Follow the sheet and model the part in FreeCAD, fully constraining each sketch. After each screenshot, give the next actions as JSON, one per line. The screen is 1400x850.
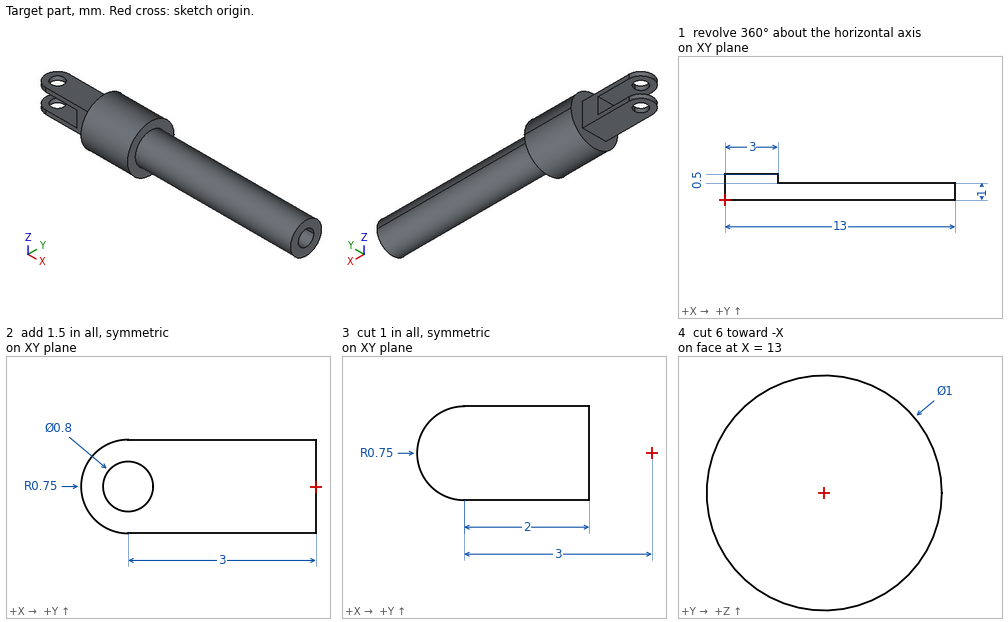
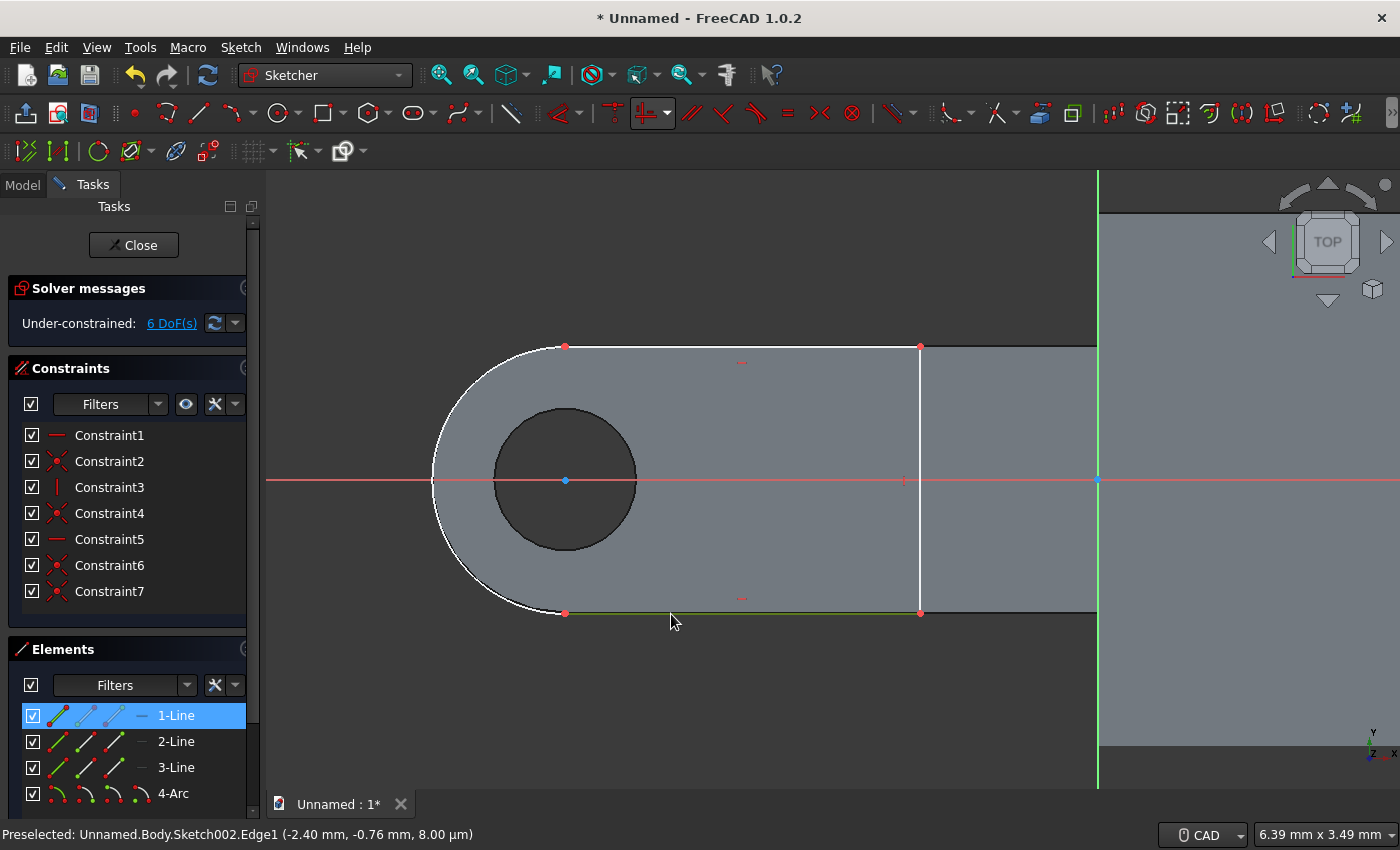
{"action": "left_click", "coordinate": [458, 402]}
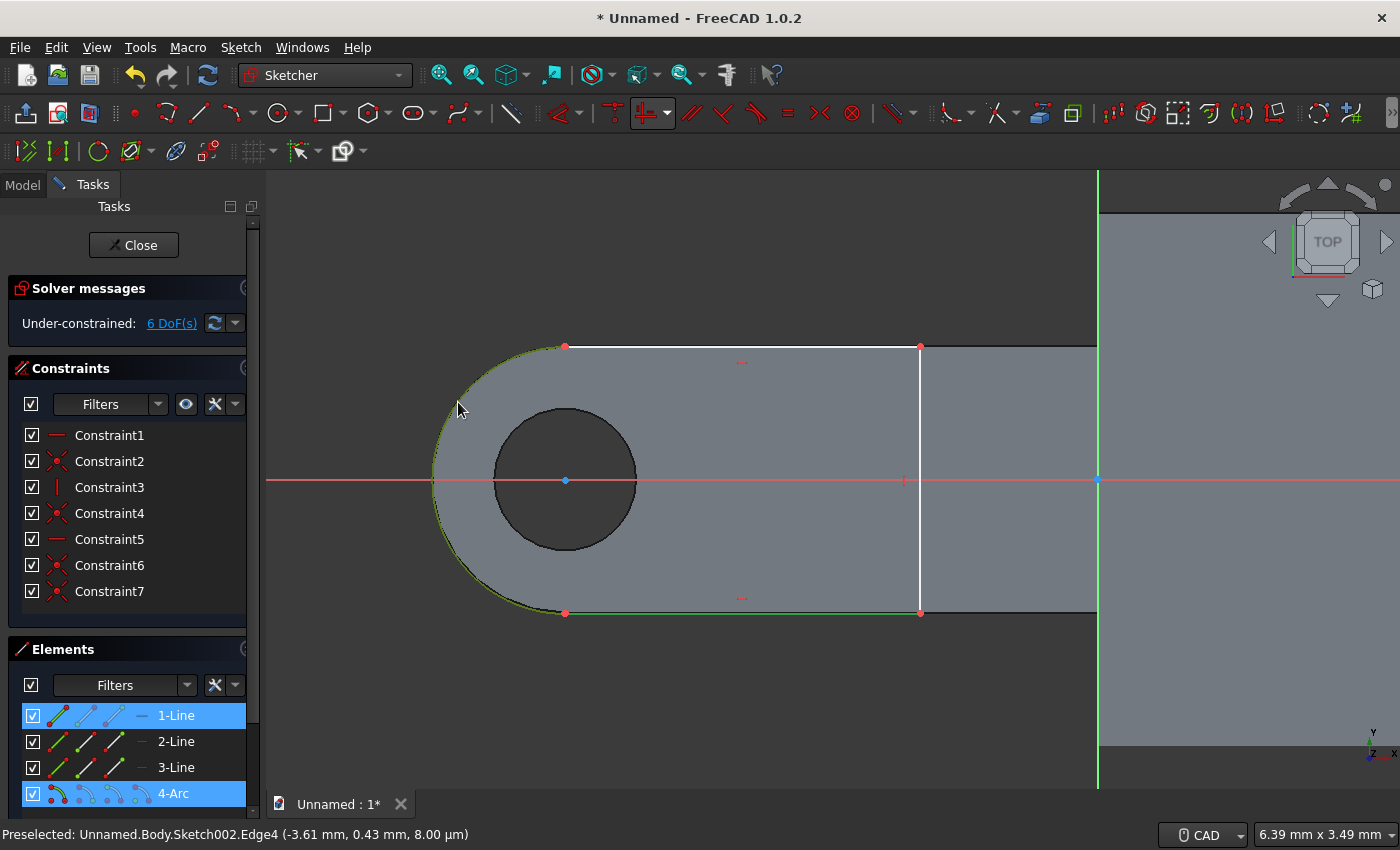
{"action": "left_click", "coordinate": [756, 114]}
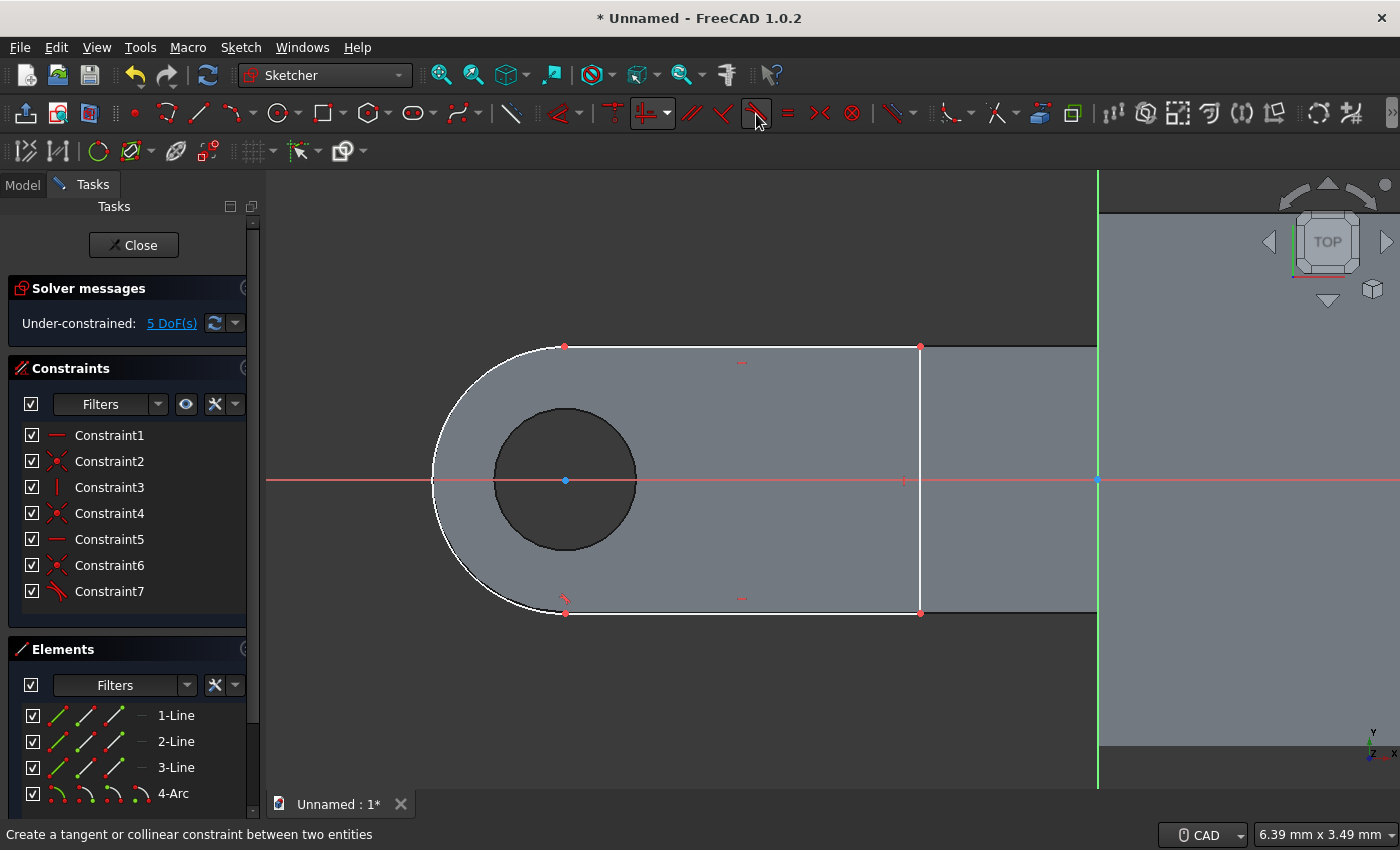
{"action": "left_click", "coordinate": [814, 347]}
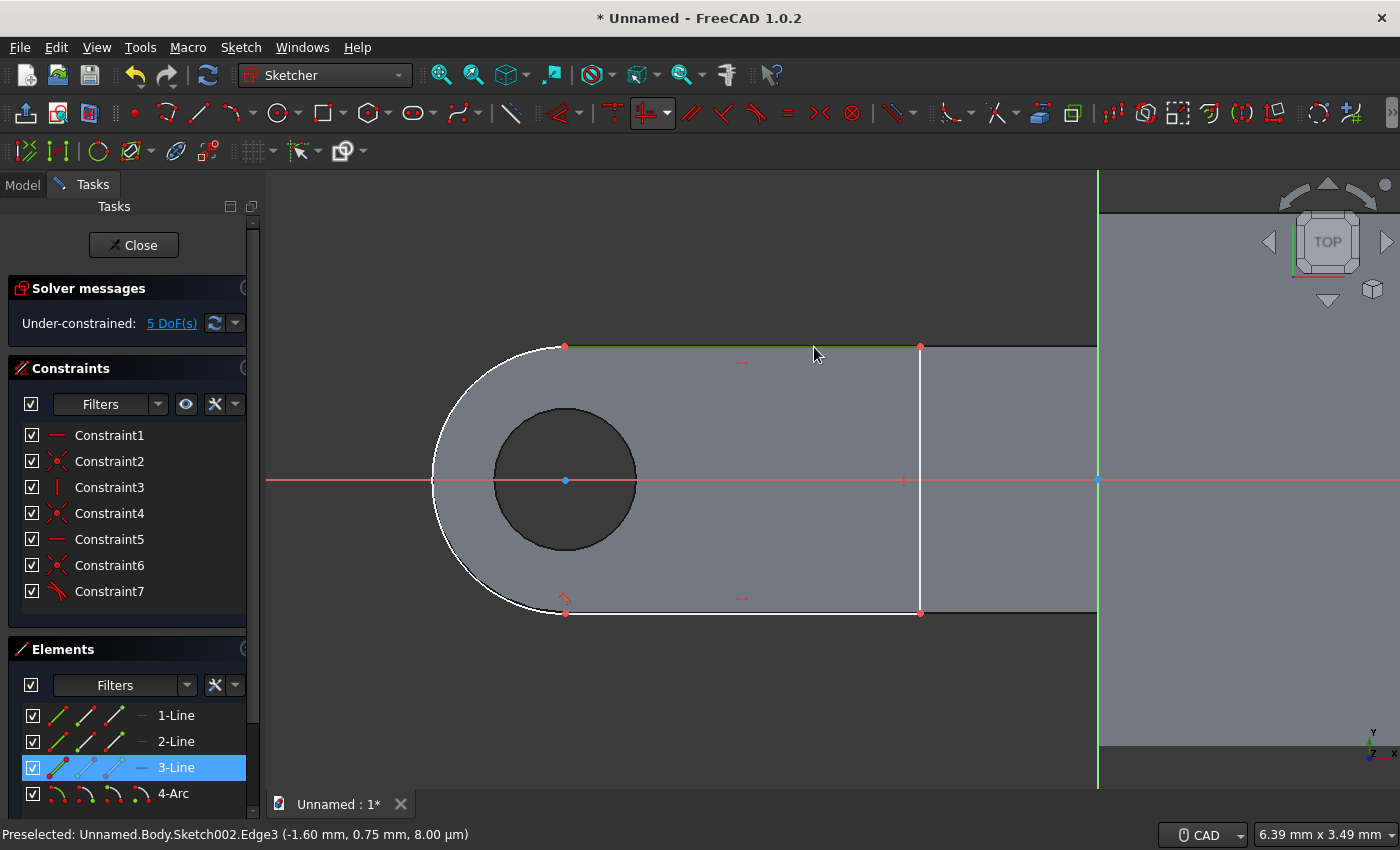
{"action": "left_click", "coordinate": [458, 403]}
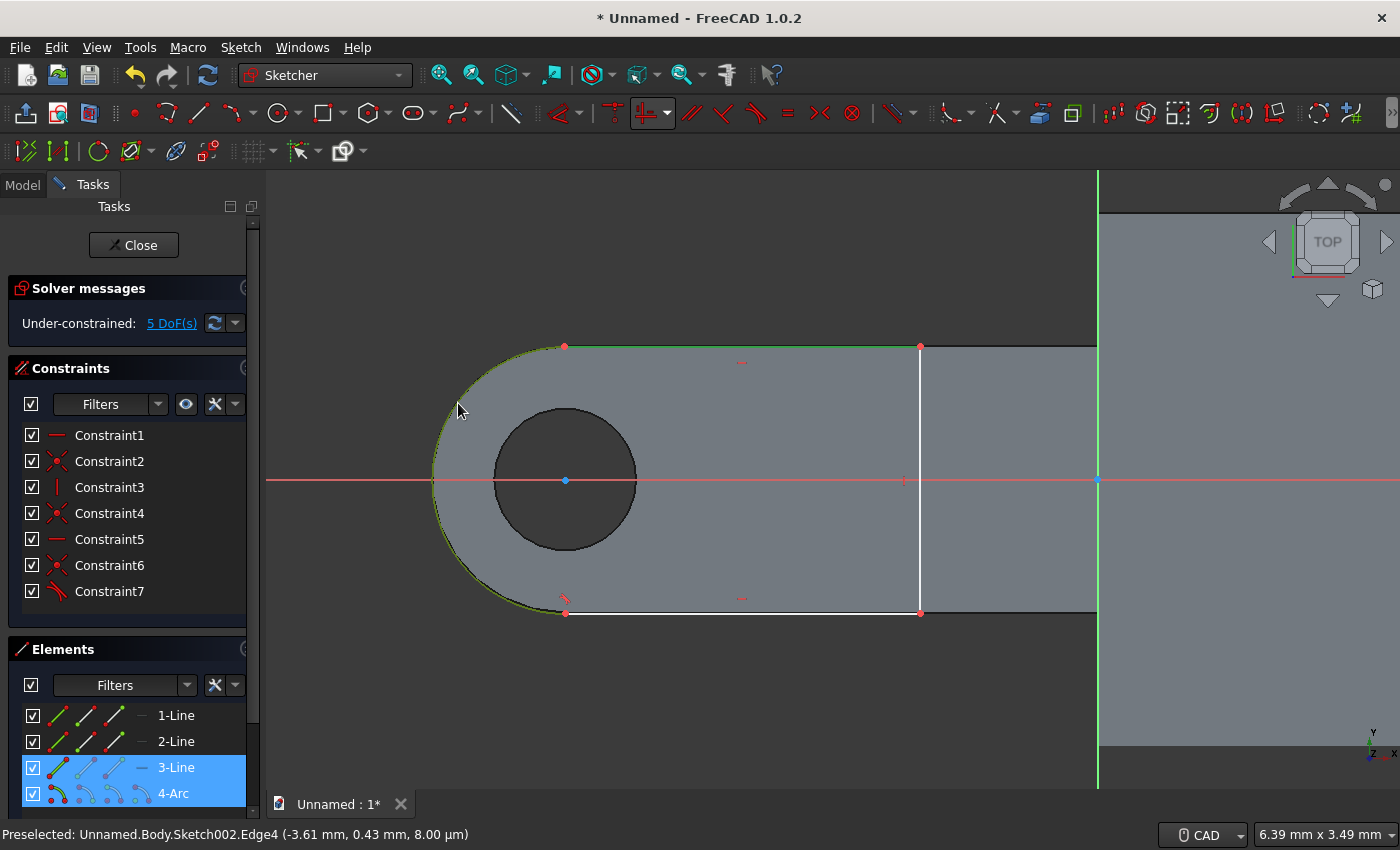
{"action": "left_click", "coordinate": [756, 114]}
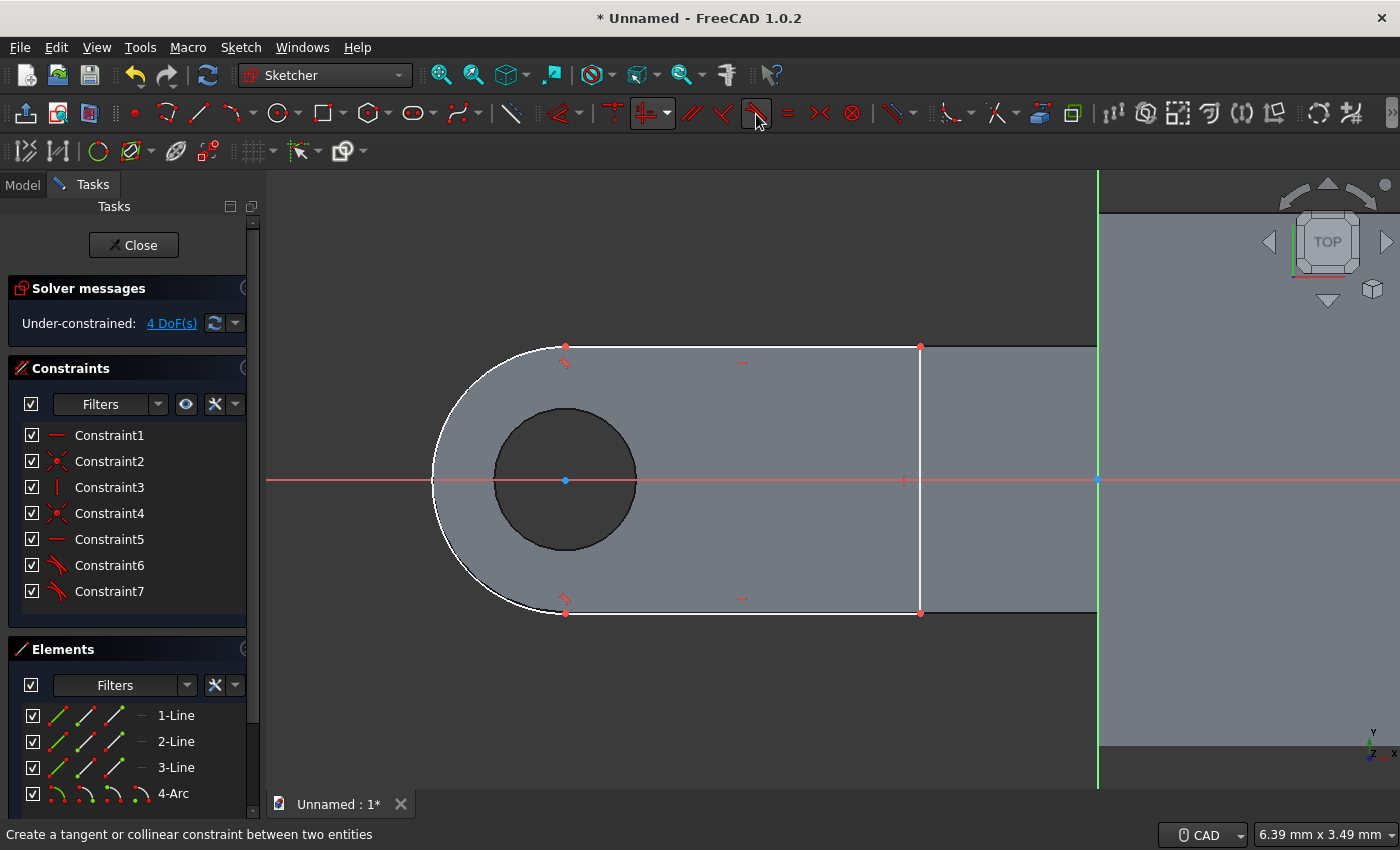
{"action": "left_click", "coordinate": [566, 480]}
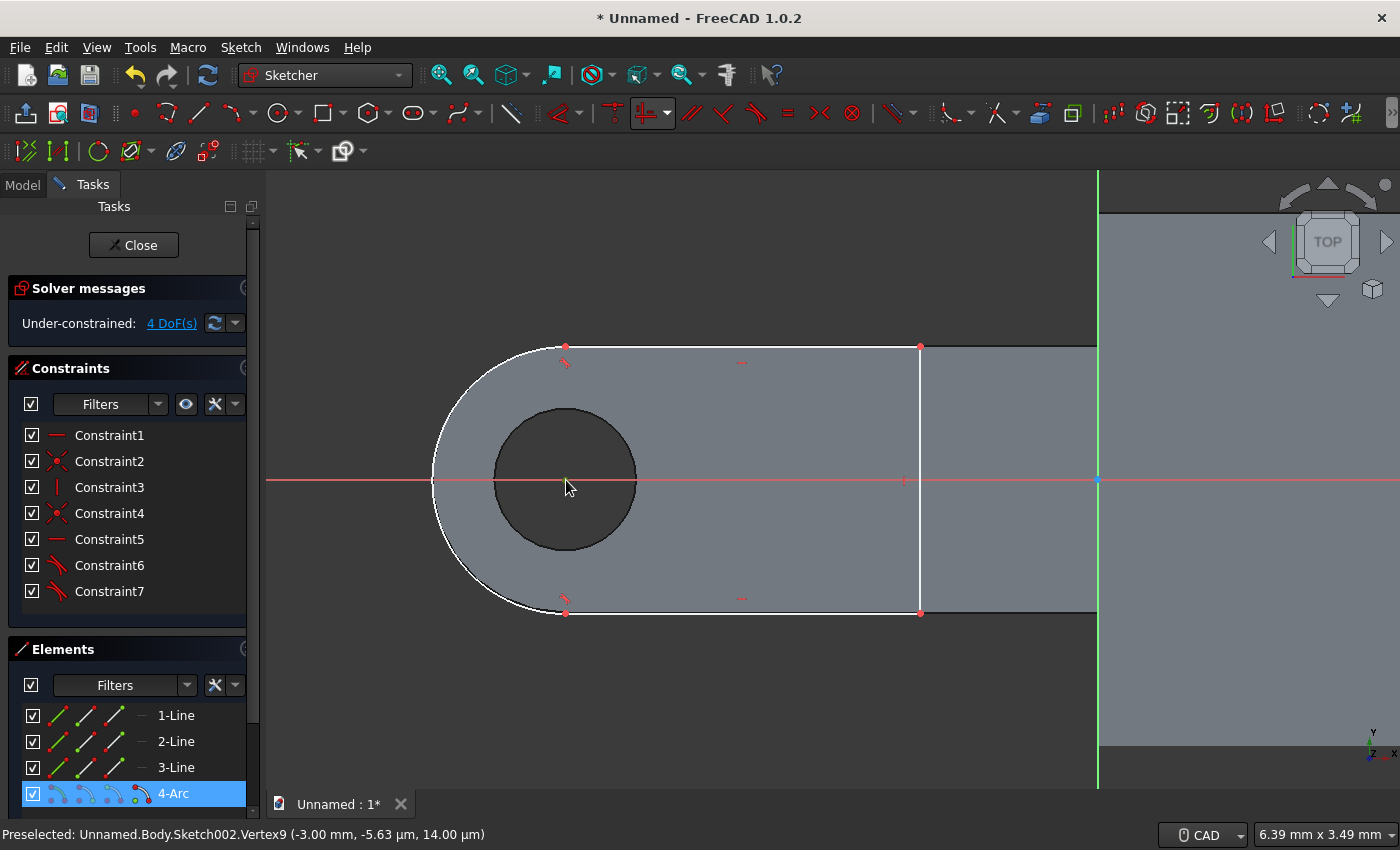
{"action": "left_click", "coordinate": [361, 480]}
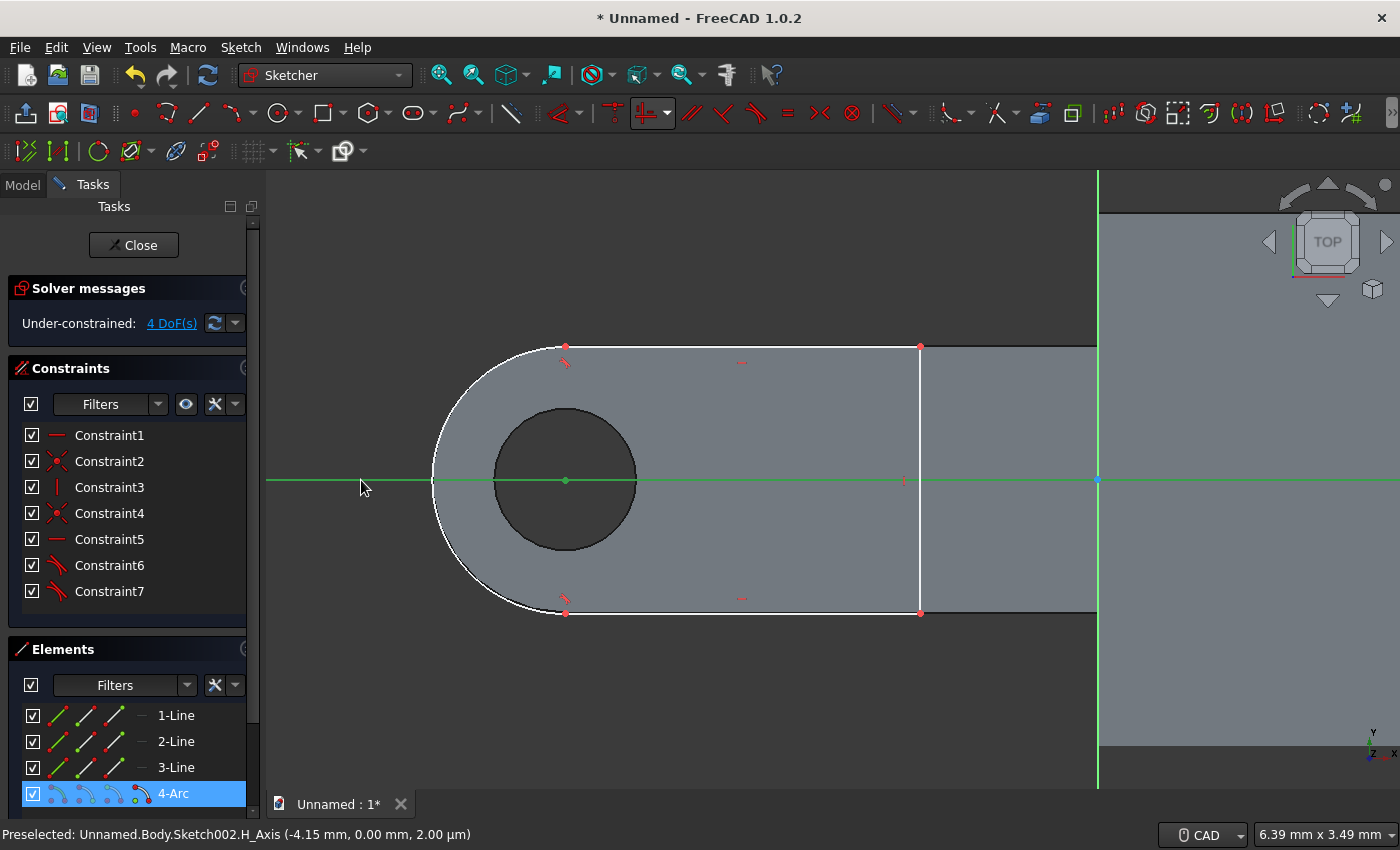
{"action": "left_click", "coordinate": [614, 114]}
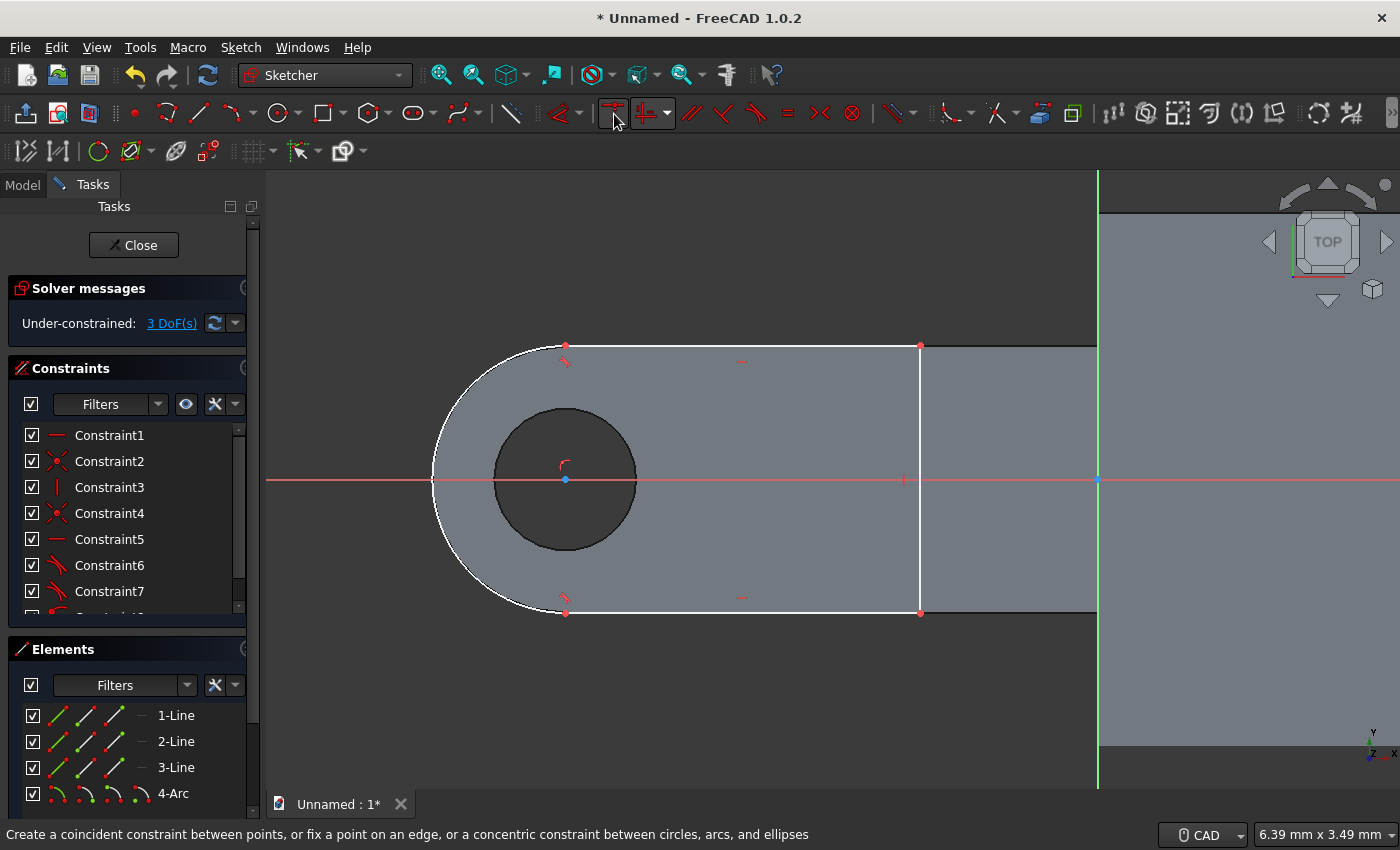
{"action": "left_click", "coordinate": [558, 114]}